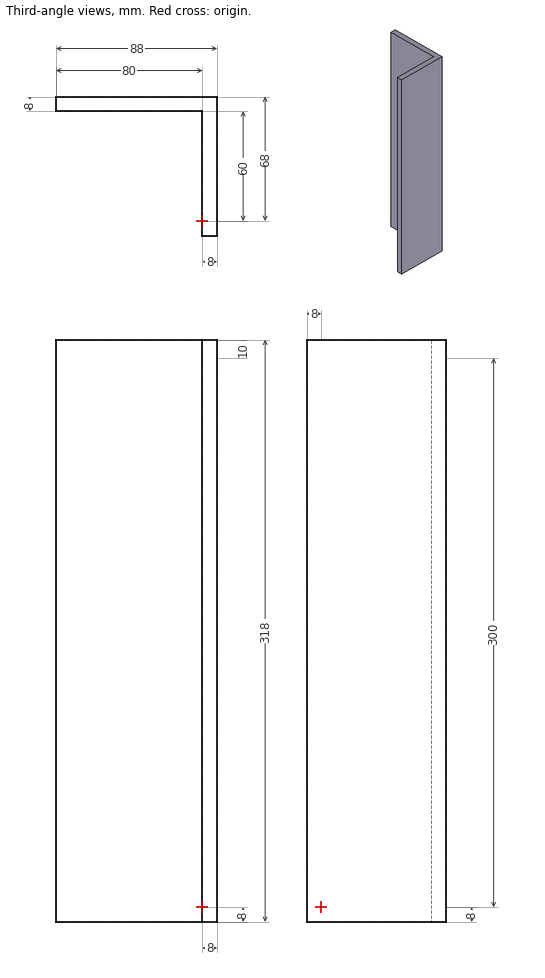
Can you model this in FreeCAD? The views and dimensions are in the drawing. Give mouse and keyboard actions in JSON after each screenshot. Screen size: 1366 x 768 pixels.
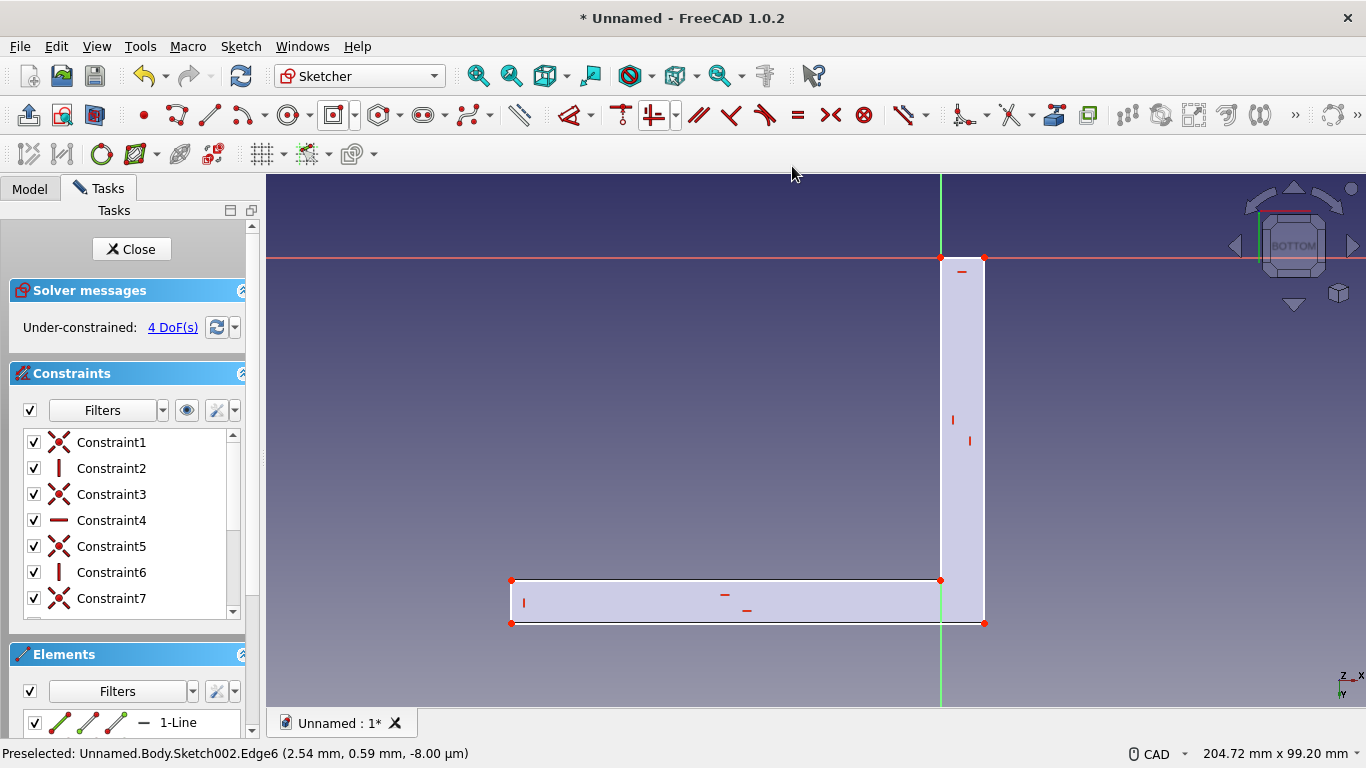
{"action": "left_click", "coordinate": [568, 116]}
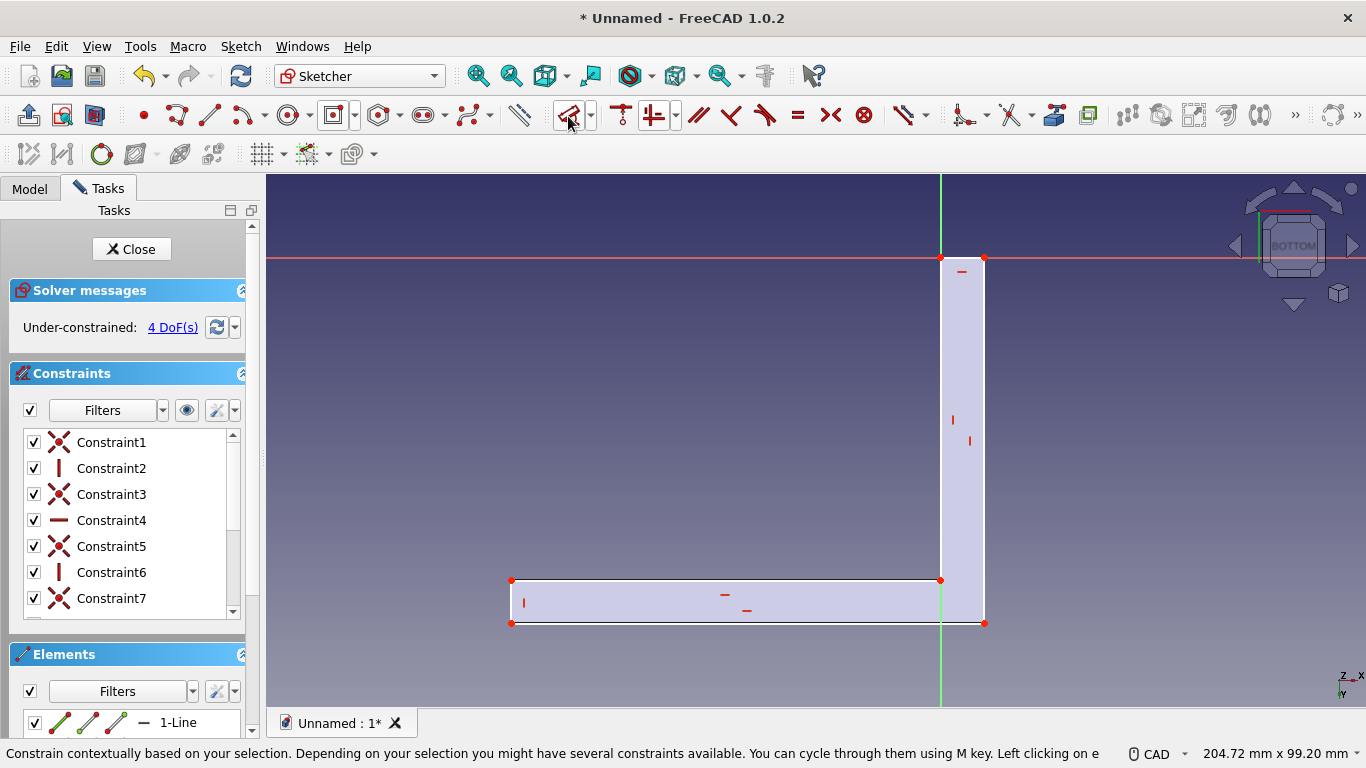
{"action": "left_click", "coordinate": [511, 594]}
{"action": "left_click", "coordinate": [477, 603]}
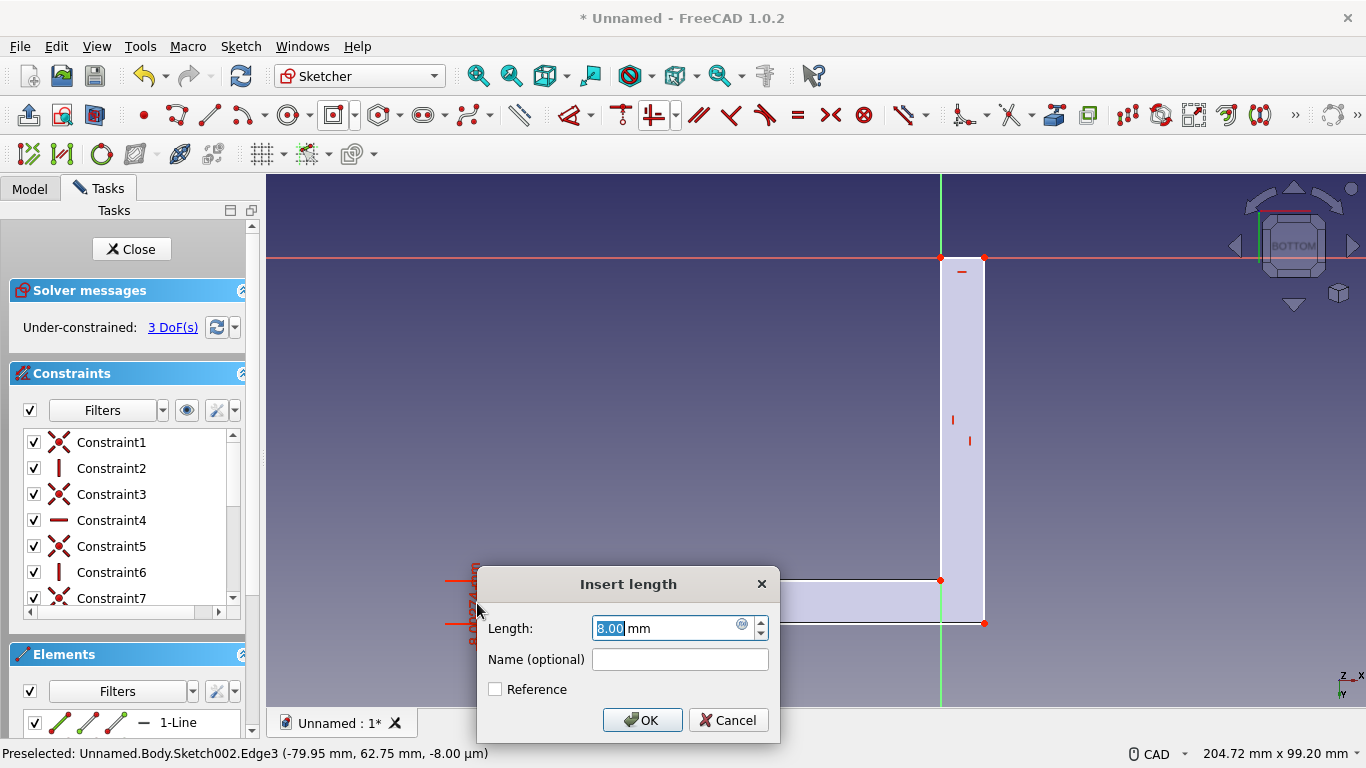
{"action": "type", "text": "8"}
{"action": "key", "text": "Return"}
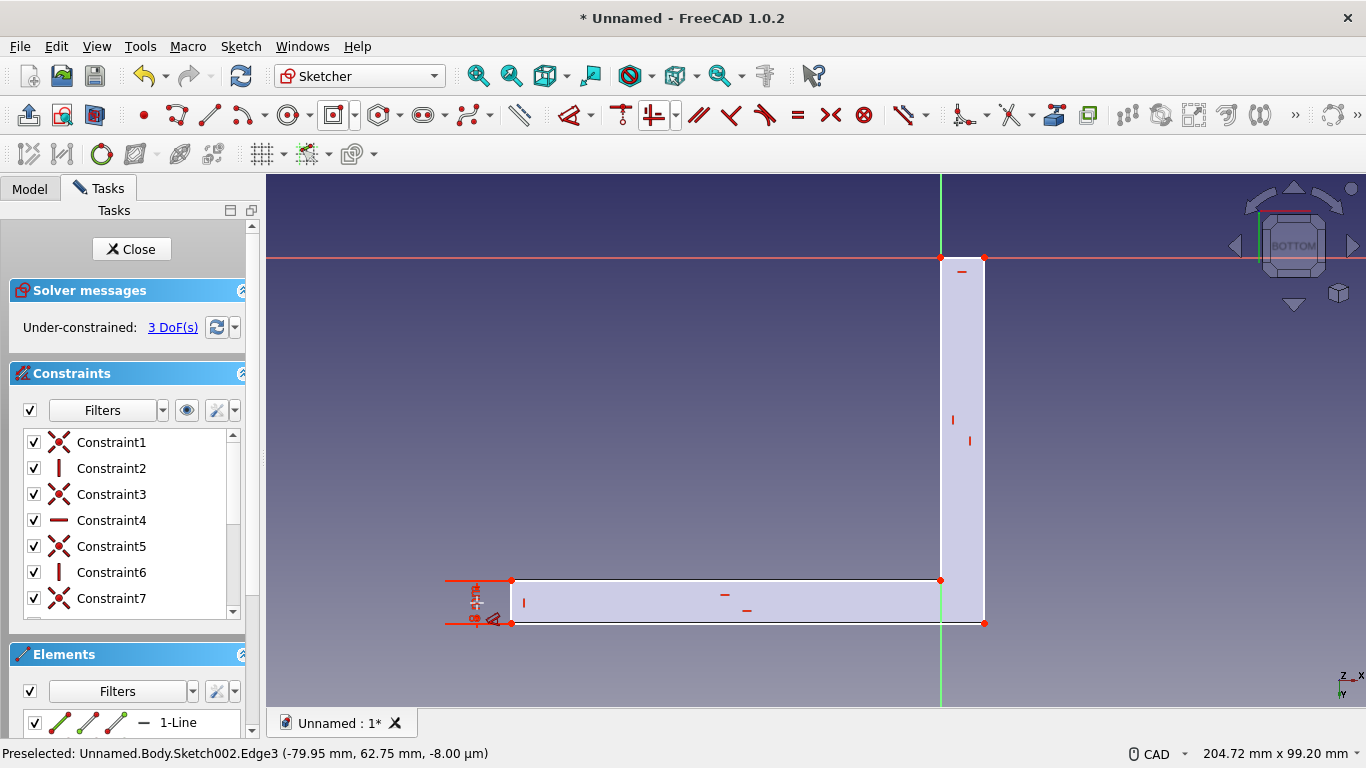
{"action": "left_click", "coordinate": [971, 258]}
{"action": "left_click", "coordinate": [962, 224]}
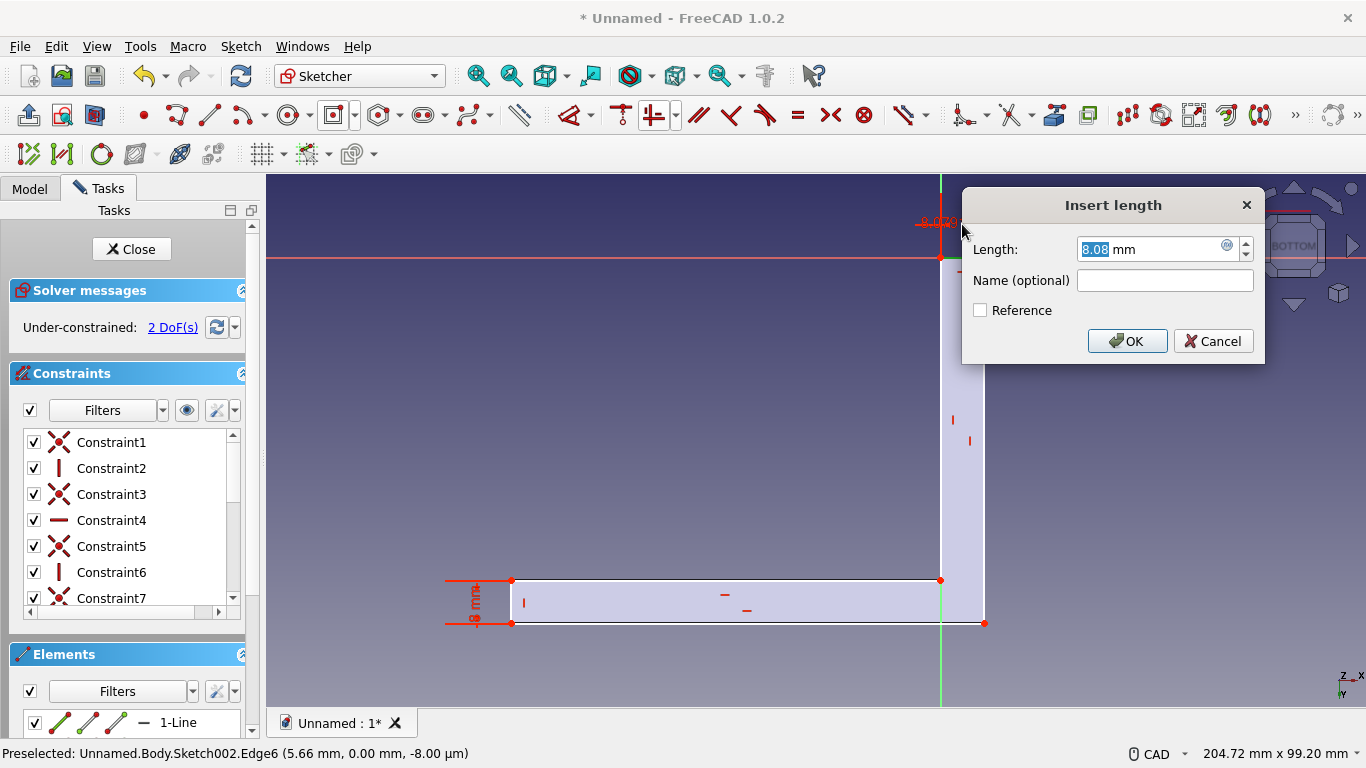
{"action": "type", "text": "8"}
{"action": "key", "text": "Return"}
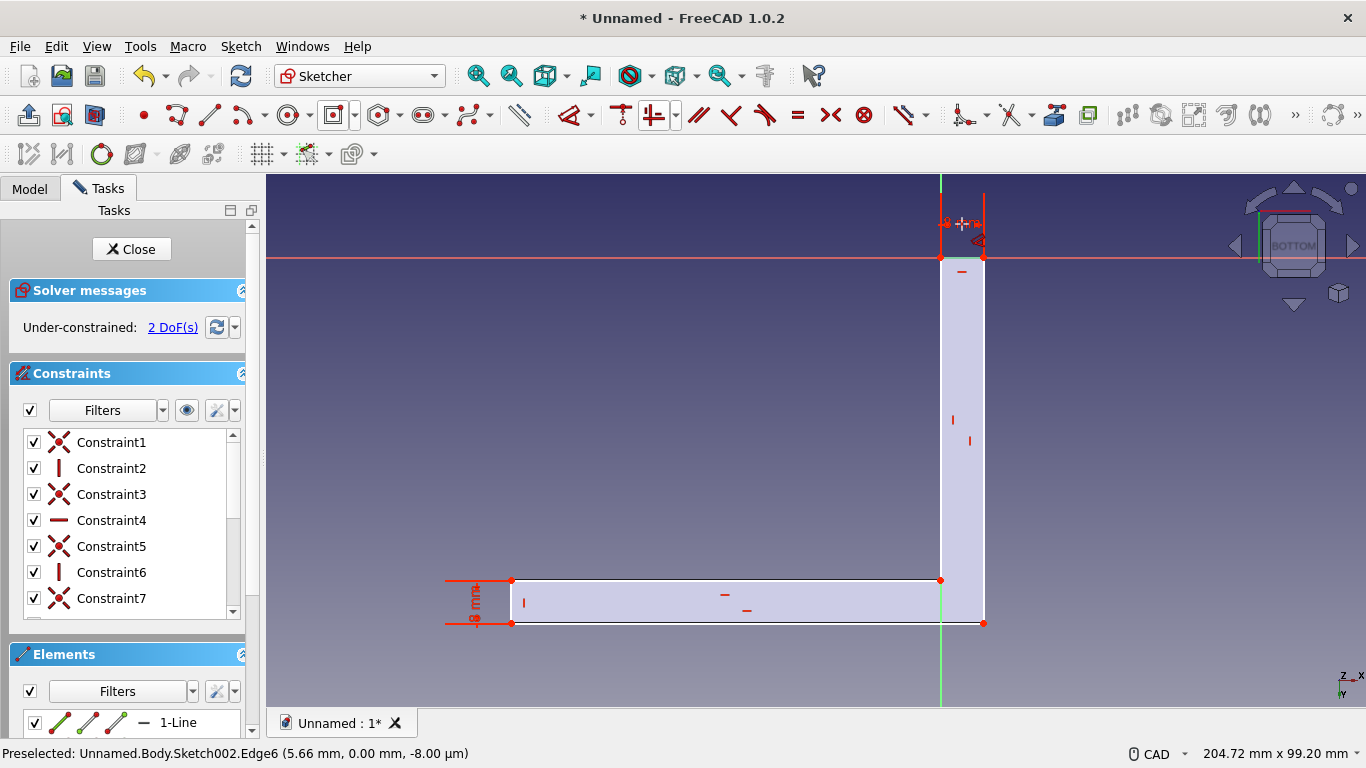
{"action": "left_click", "coordinate": [941, 355]}
{"action": "left_click", "coordinate": [907, 419]}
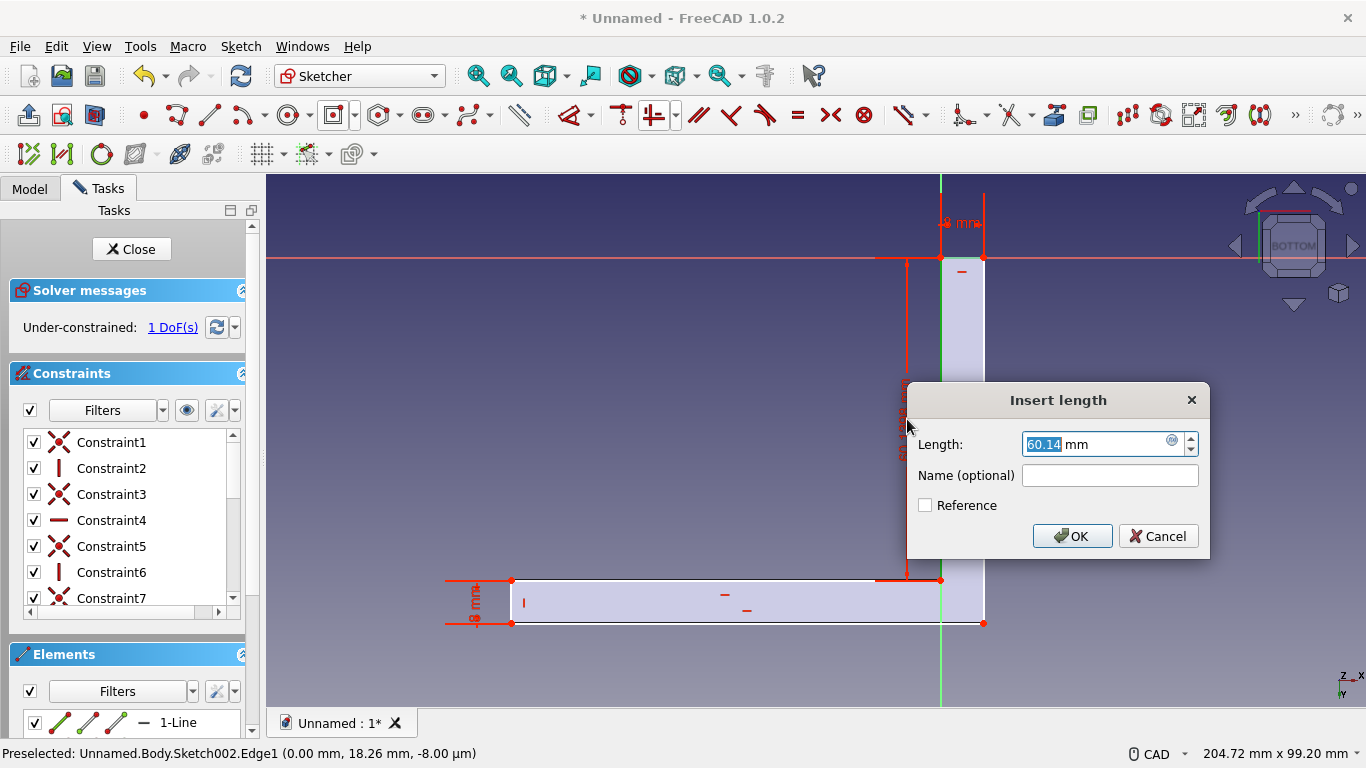
{"action": "type", "text": "60"}
{"action": "key", "text": "Return"}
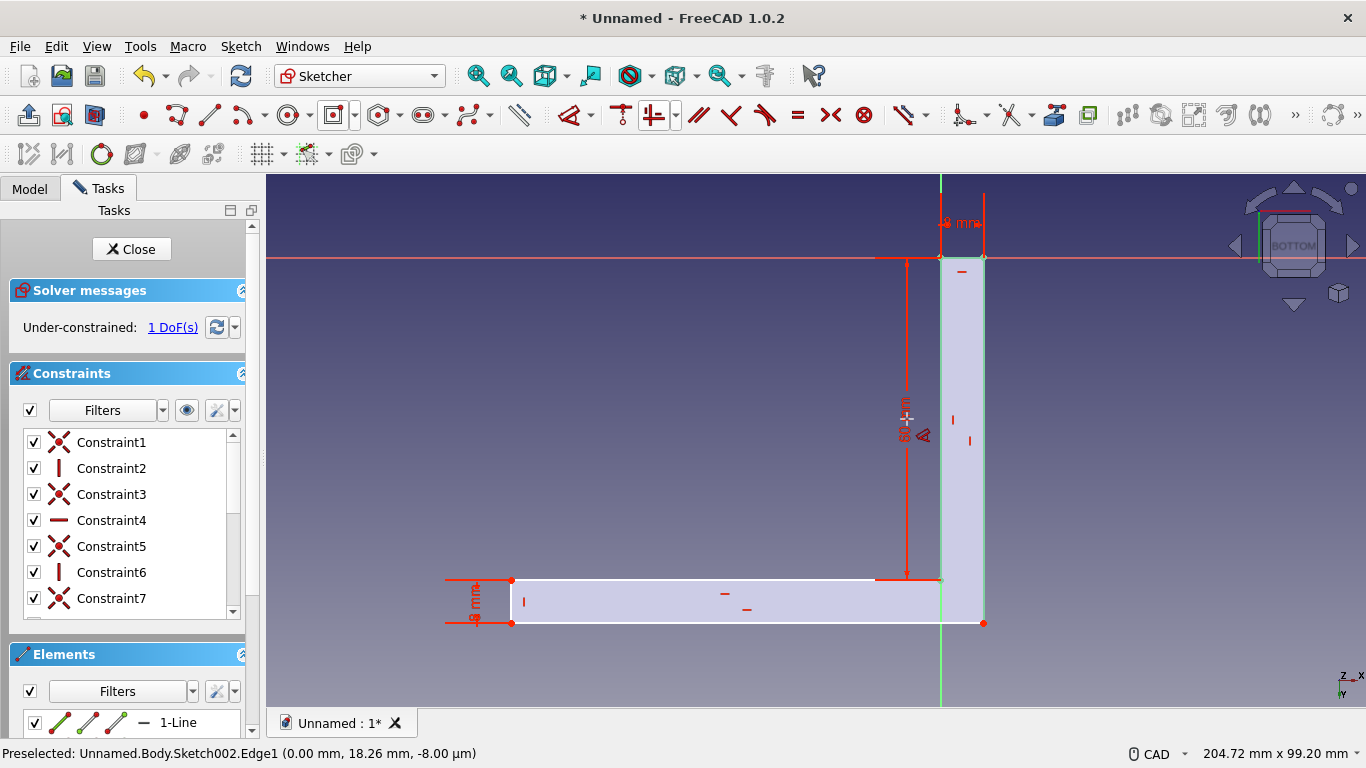
{"action": "left_click", "coordinate": [812, 580]}
{"action": "left_click", "coordinate": [726, 546]}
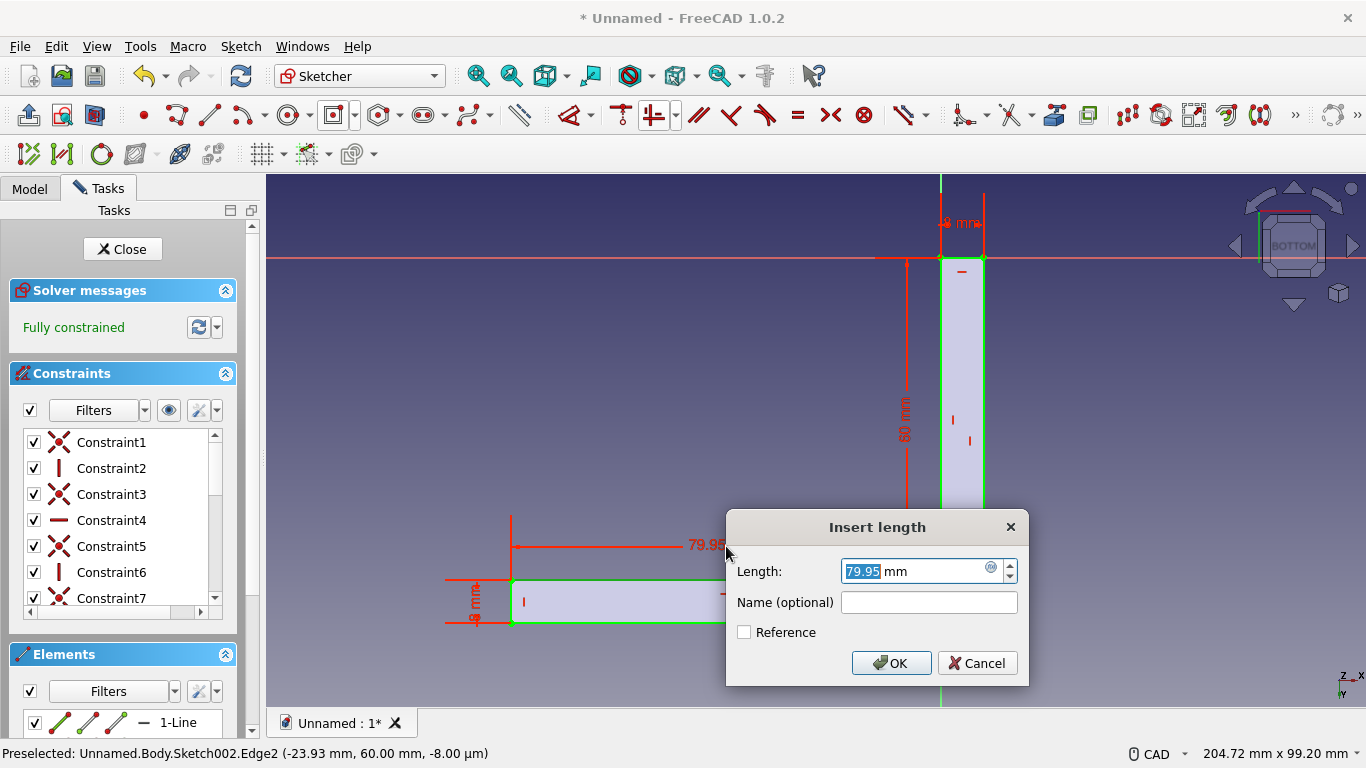
{"action": "type", "text": "80"}
{"action": "key", "text": "Return"}
{"action": "key", "text": "Escape"}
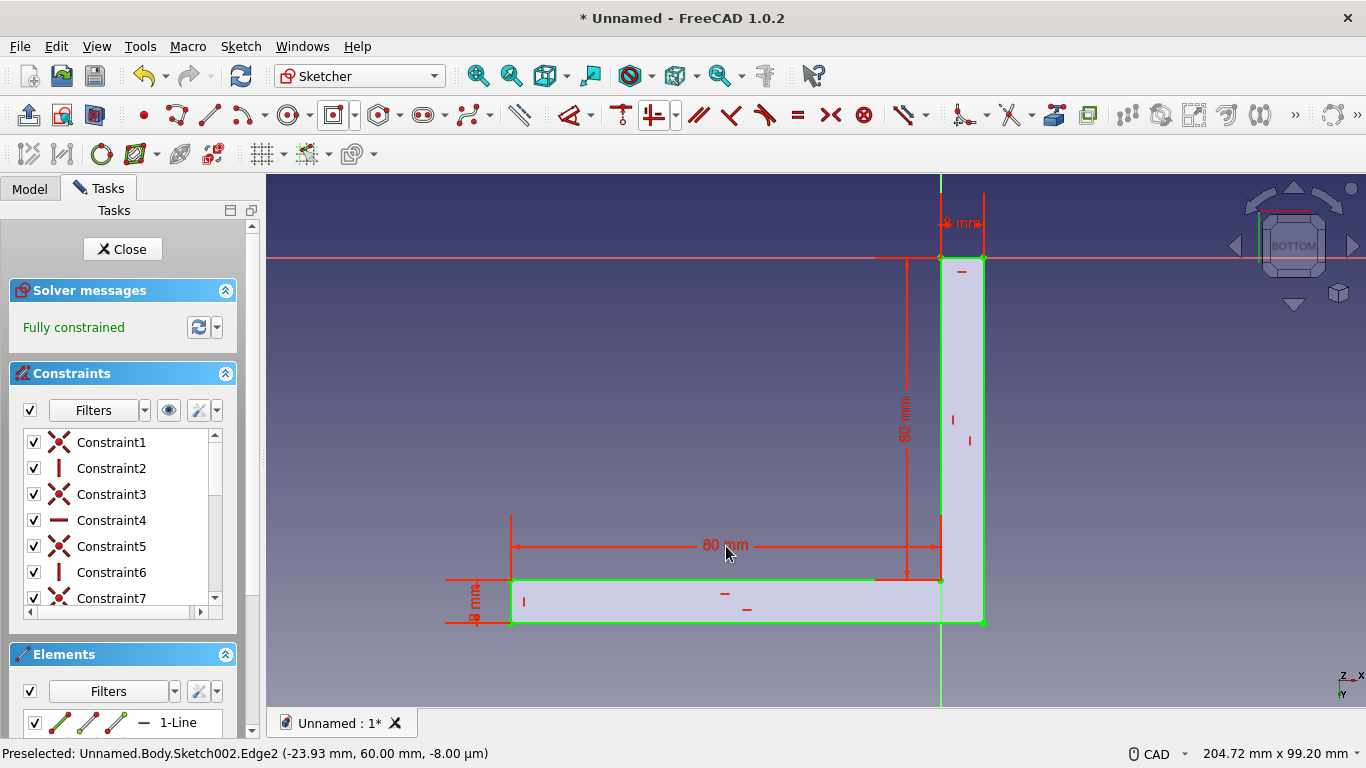
{"action": "left_click", "coordinate": [123, 249]}